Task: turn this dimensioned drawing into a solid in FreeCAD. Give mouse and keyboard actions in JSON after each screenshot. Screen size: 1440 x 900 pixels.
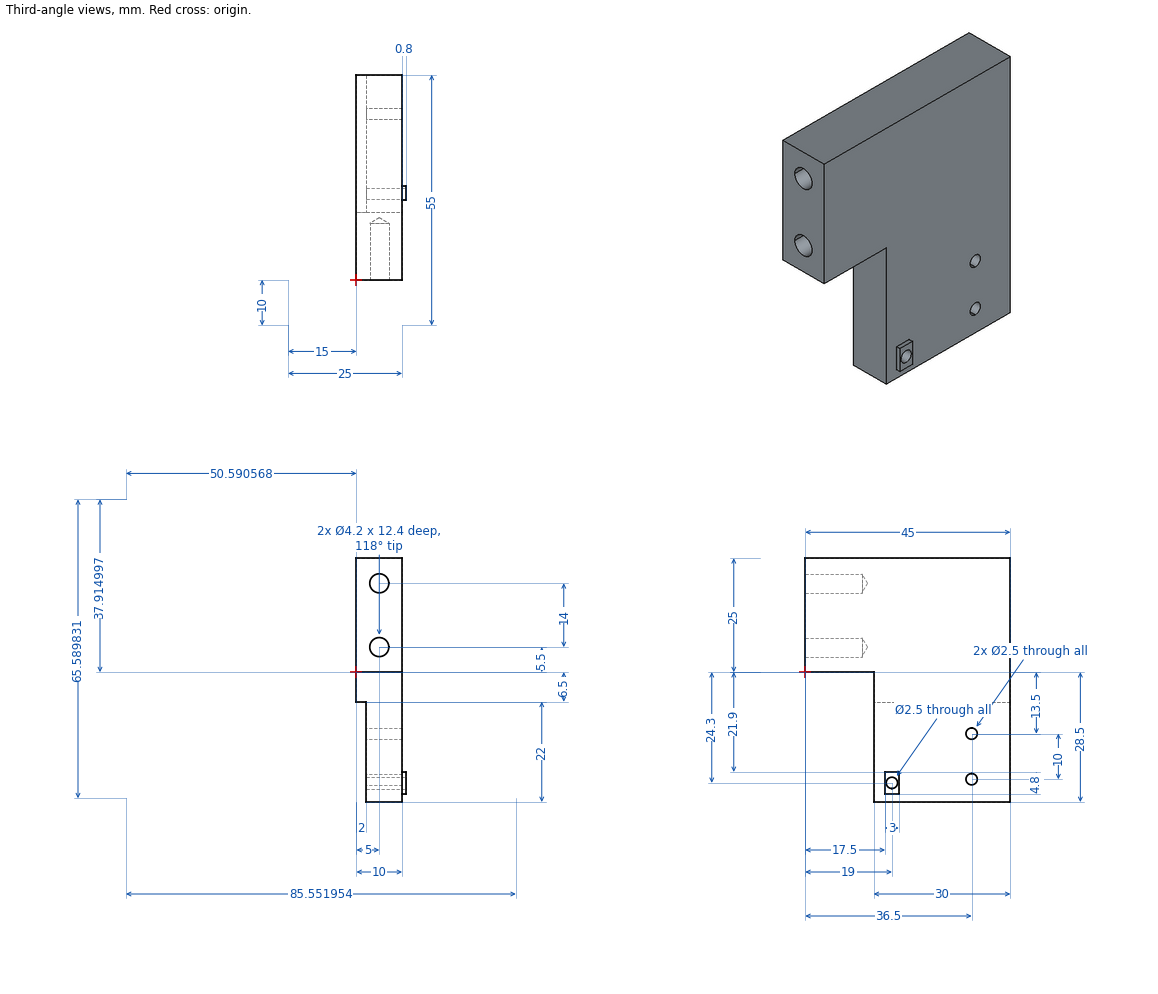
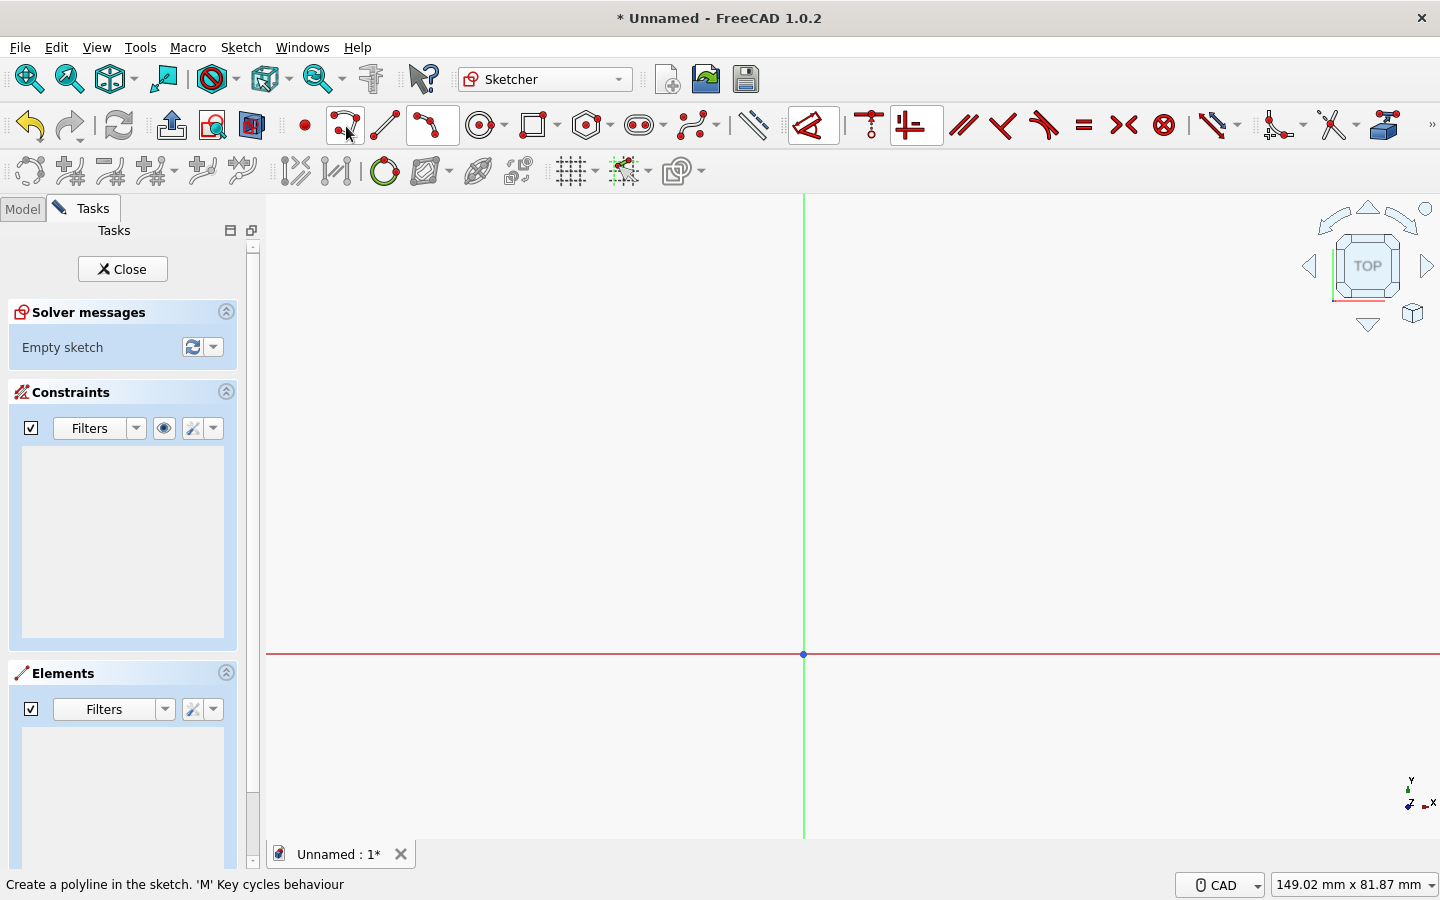
{"action": "left_click", "coordinate": [804, 654]}
{"action": "left_click", "coordinate": [686, 645]}
{"action": "left_click", "coordinate": [686, 733]}
{"action": "left_click", "coordinate": [883, 733]}
{"action": "left_click", "coordinate": [883, 300]}
{"action": "left_click", "coordinate": [795, 300]}
{"action": "left_click", "coordinate": [804, 654]}
{"action": "key", "text": "Escape"}
{"action": "key", "text": "Escape"}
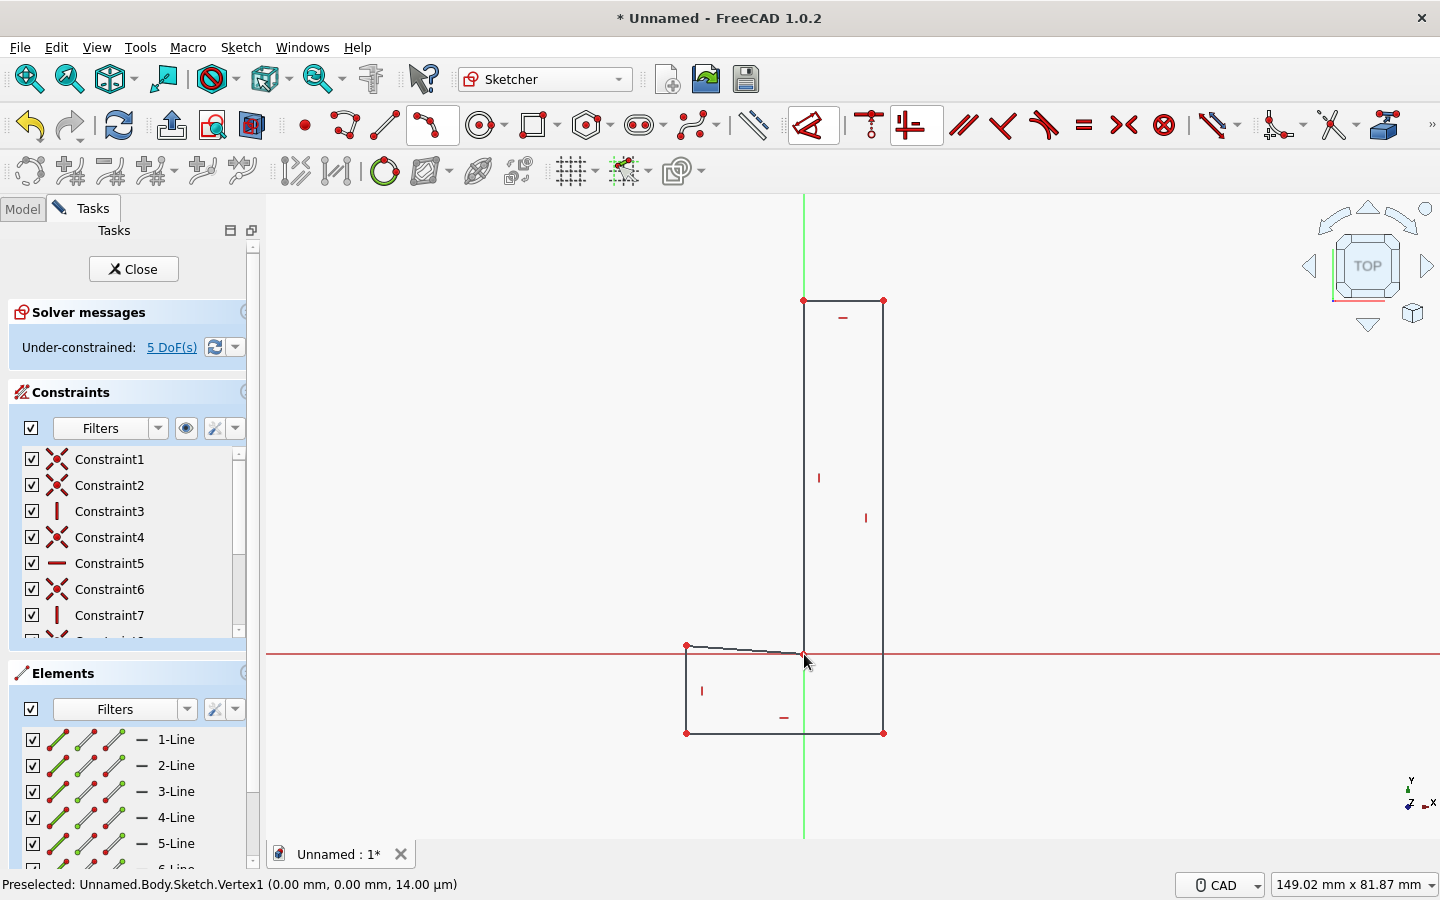
{"action": "left_click", "coordinate": [768, 652]}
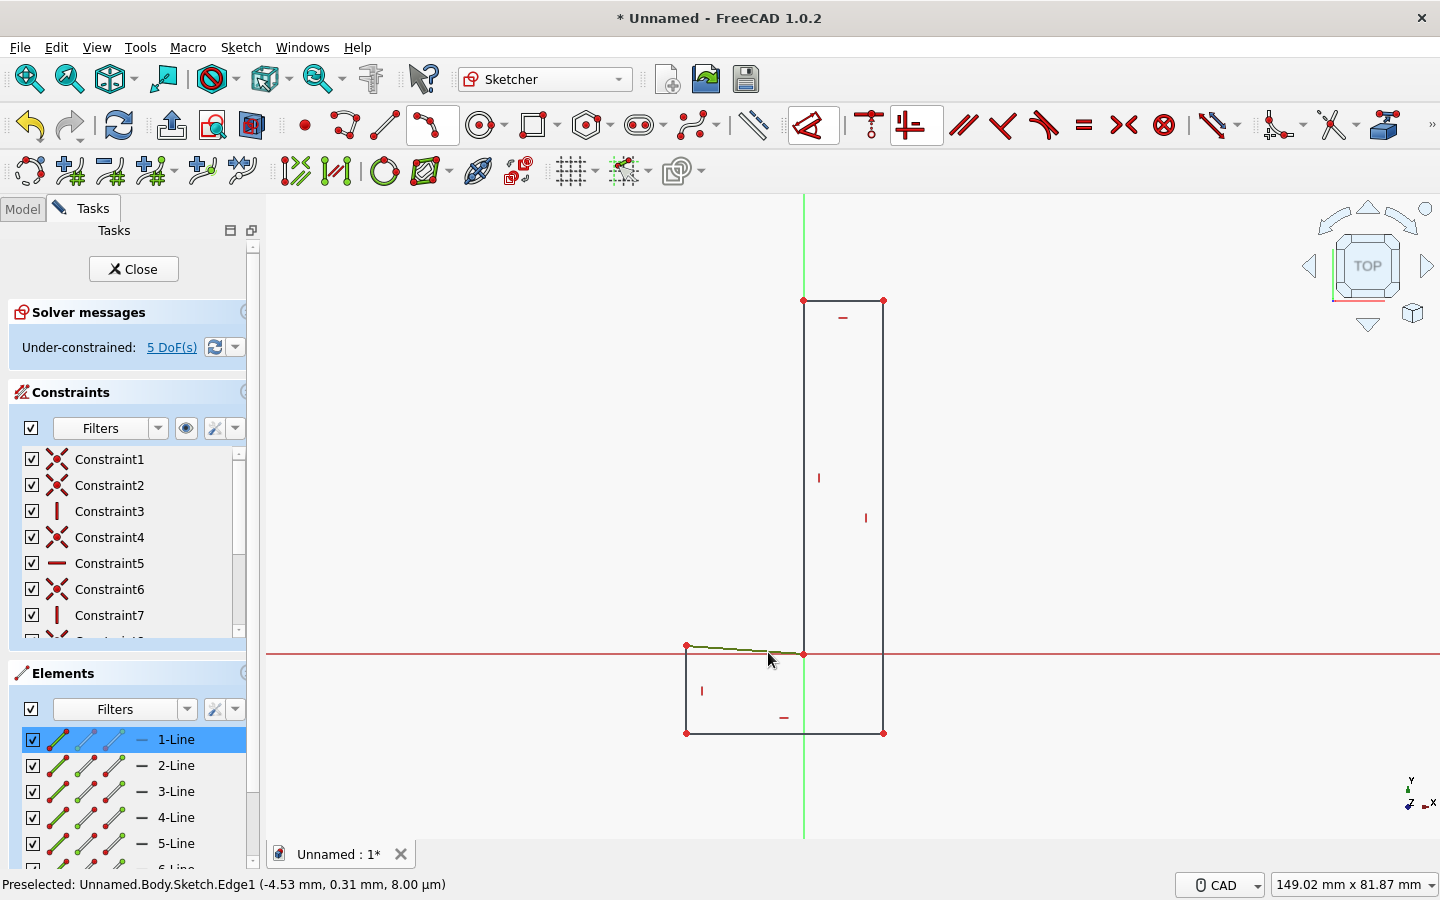
{"action": "key", "text": "h"}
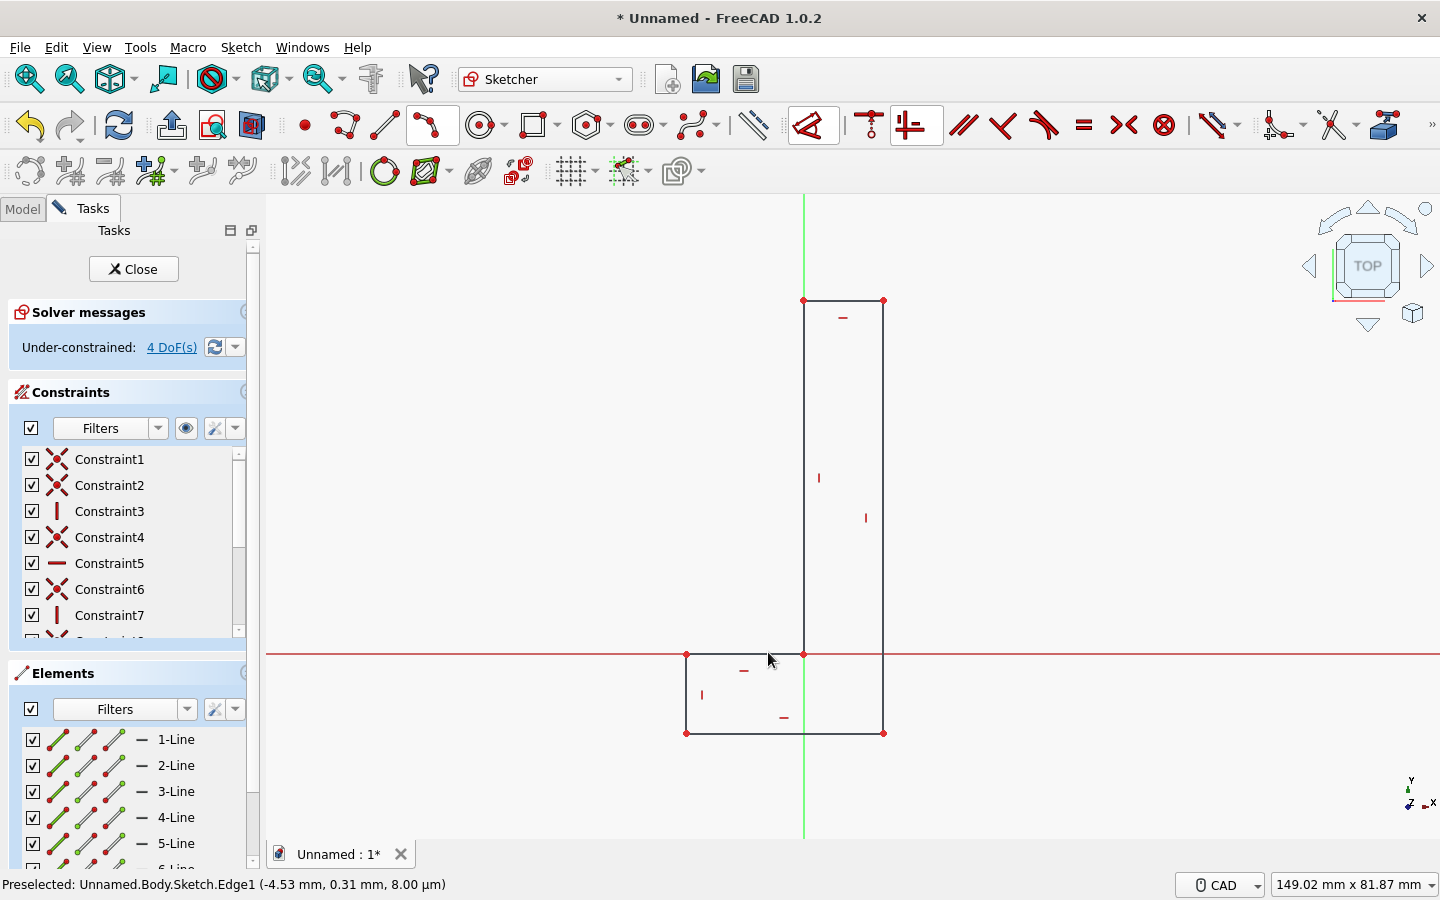
{"action": "left_click", "coordinate": [768, 654]}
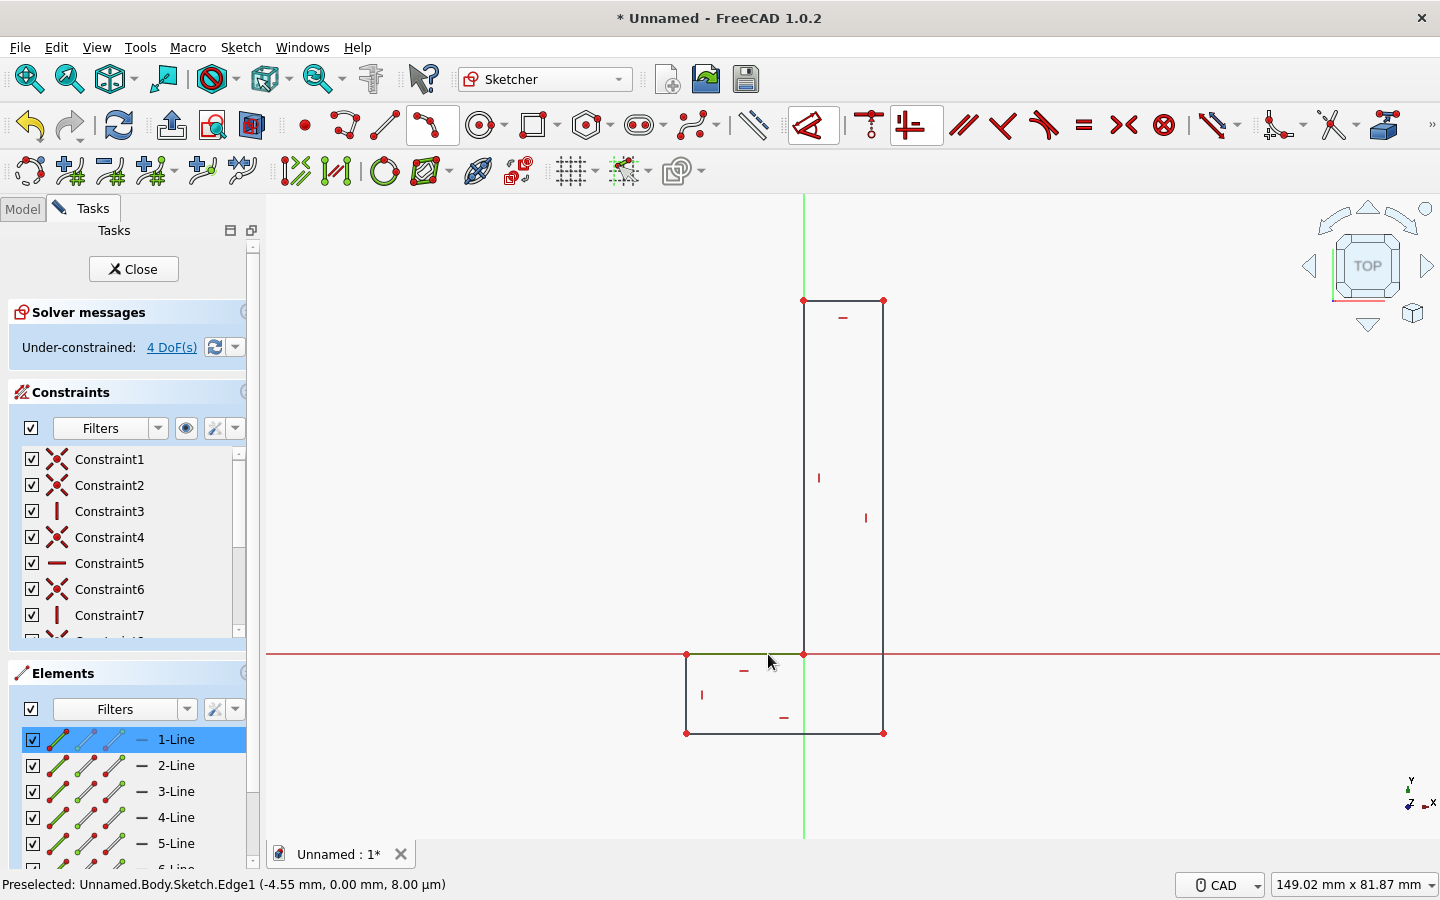
{"action": "left_click", "coordinate": [834, 126]}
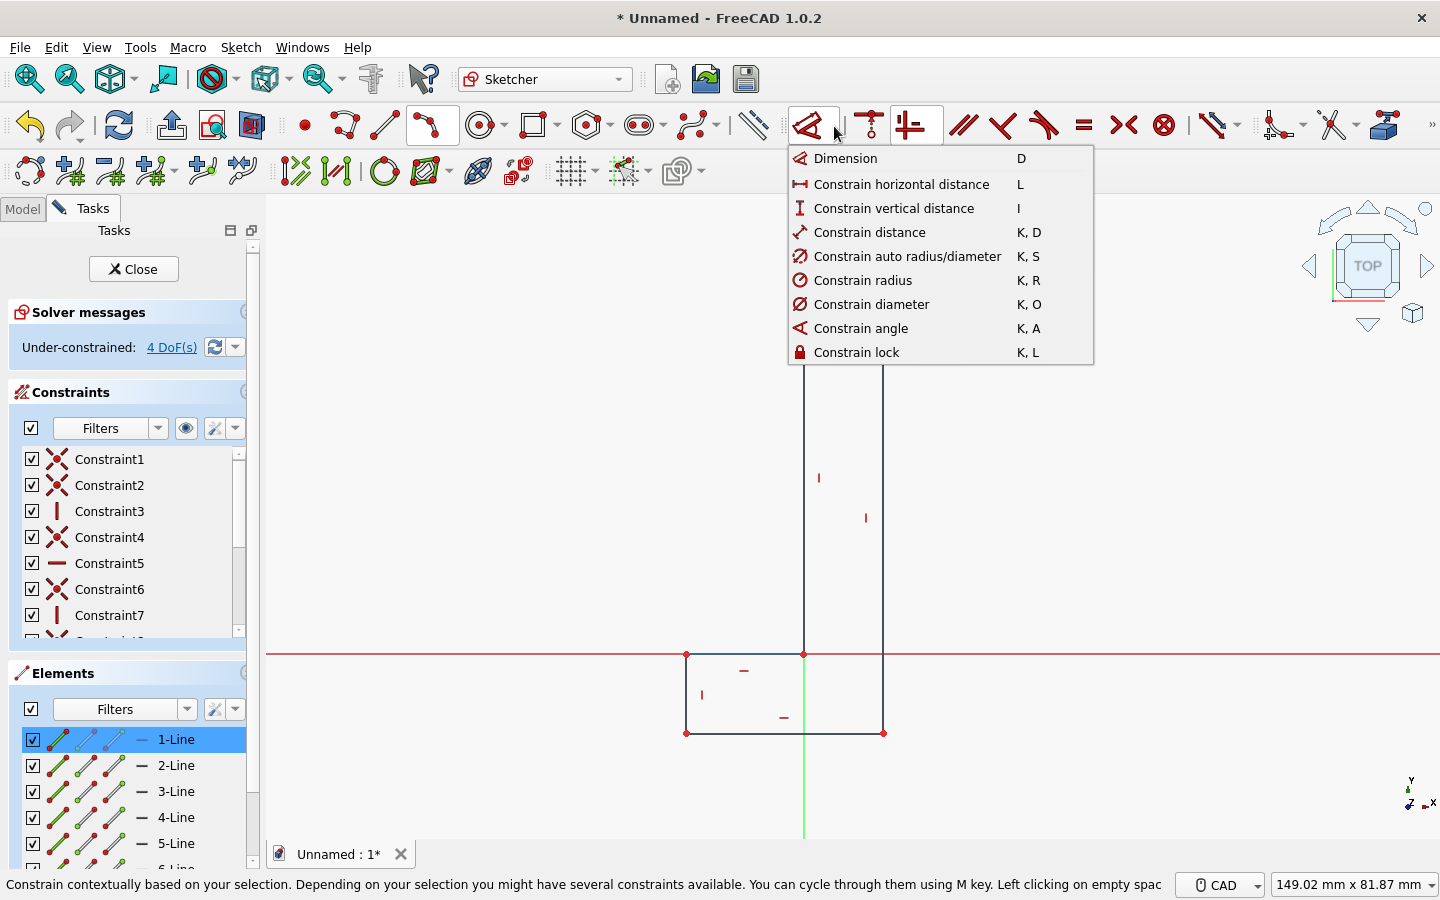
{"action": "left_click", "coordinate": [941, 184]}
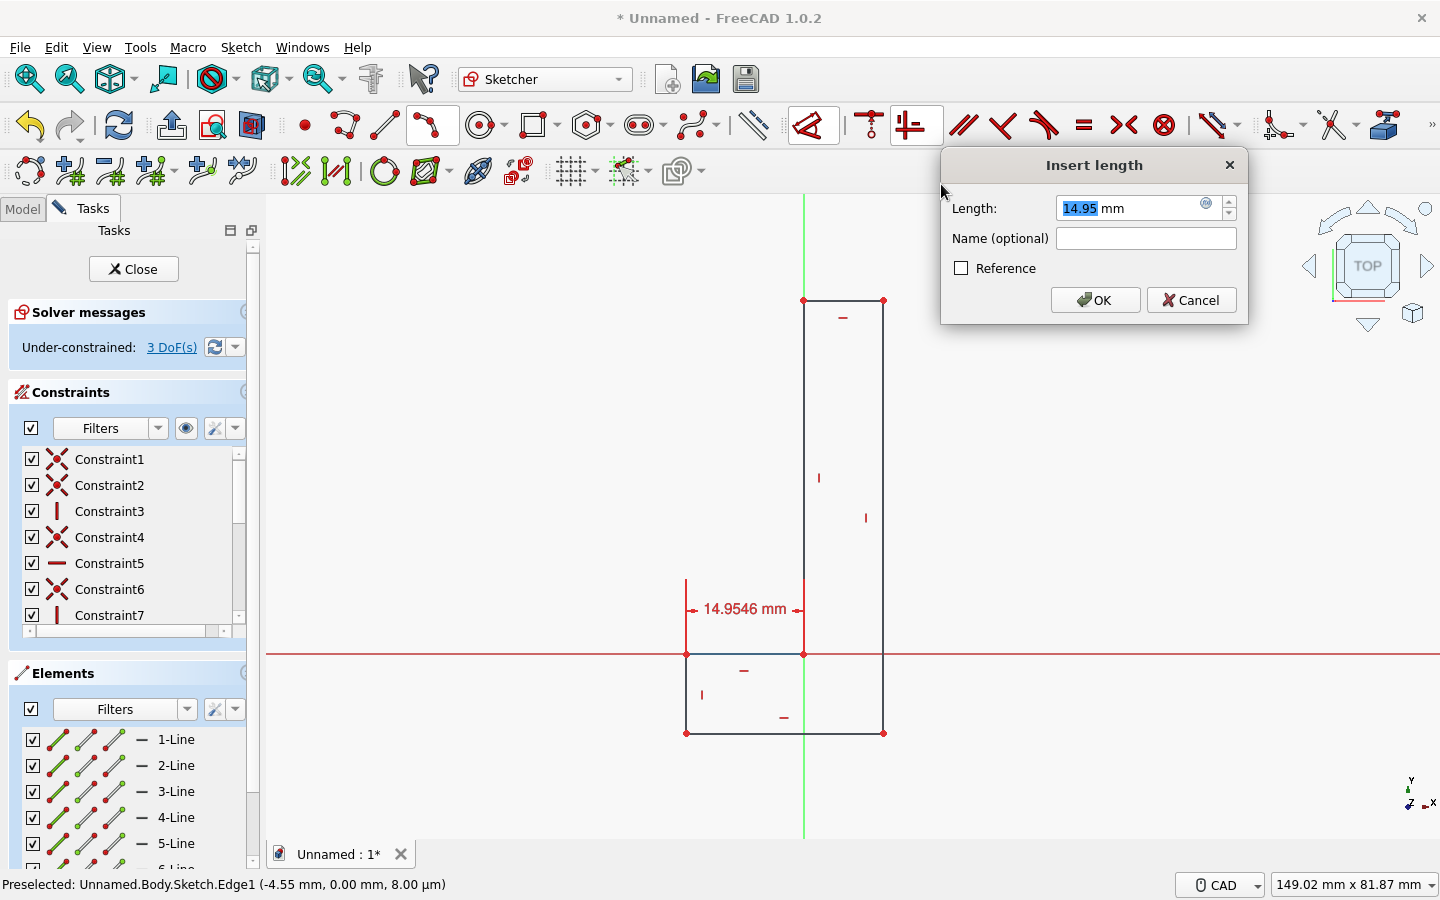
{"action": "type", "text": "15"}
{"action": "key", "text": "Return"}